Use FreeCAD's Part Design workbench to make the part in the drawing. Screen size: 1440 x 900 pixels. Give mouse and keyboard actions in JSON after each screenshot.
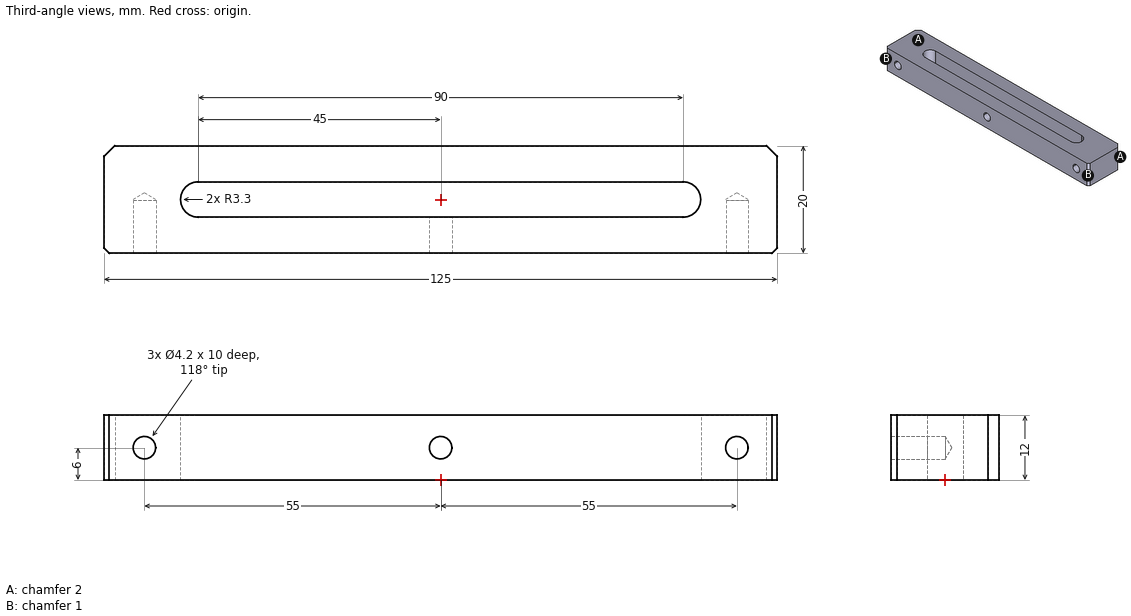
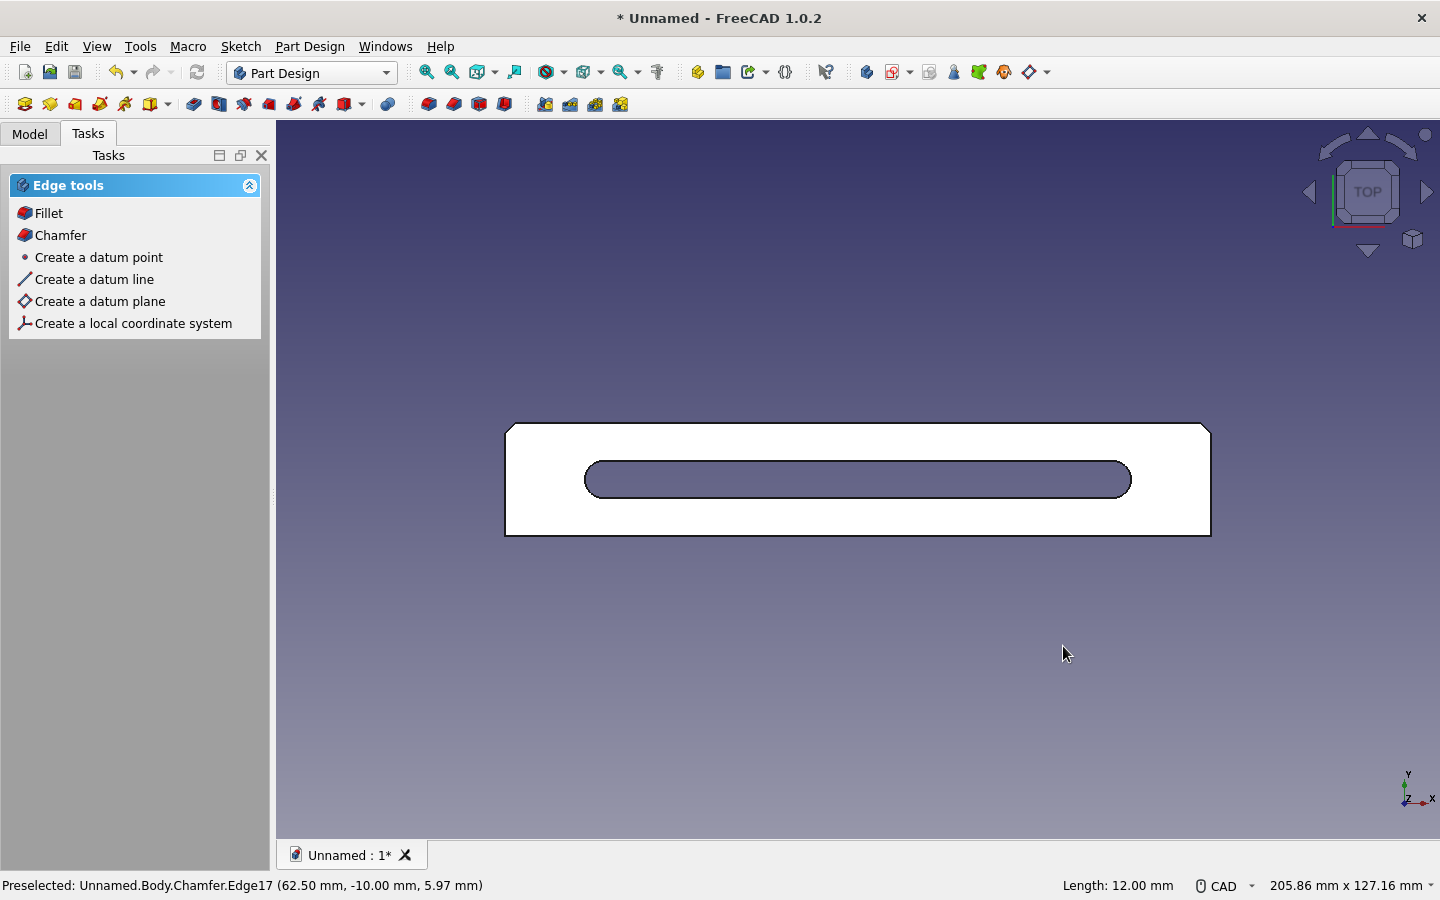
{"action": "key", "text": "1"}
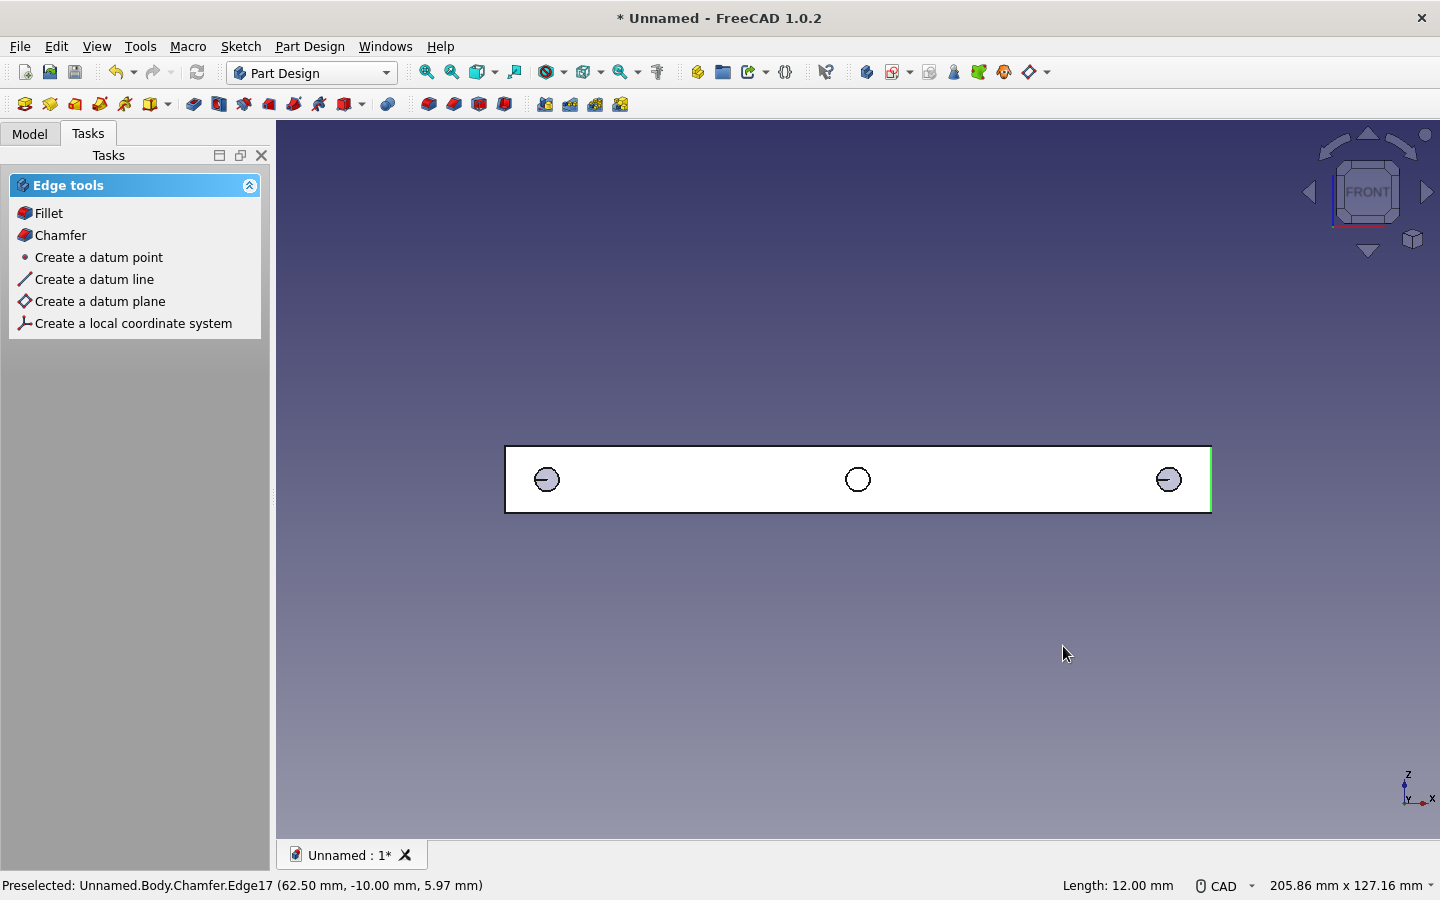
{"action": "left_click", "coordinate": [505, 479], "text": "ctrl"}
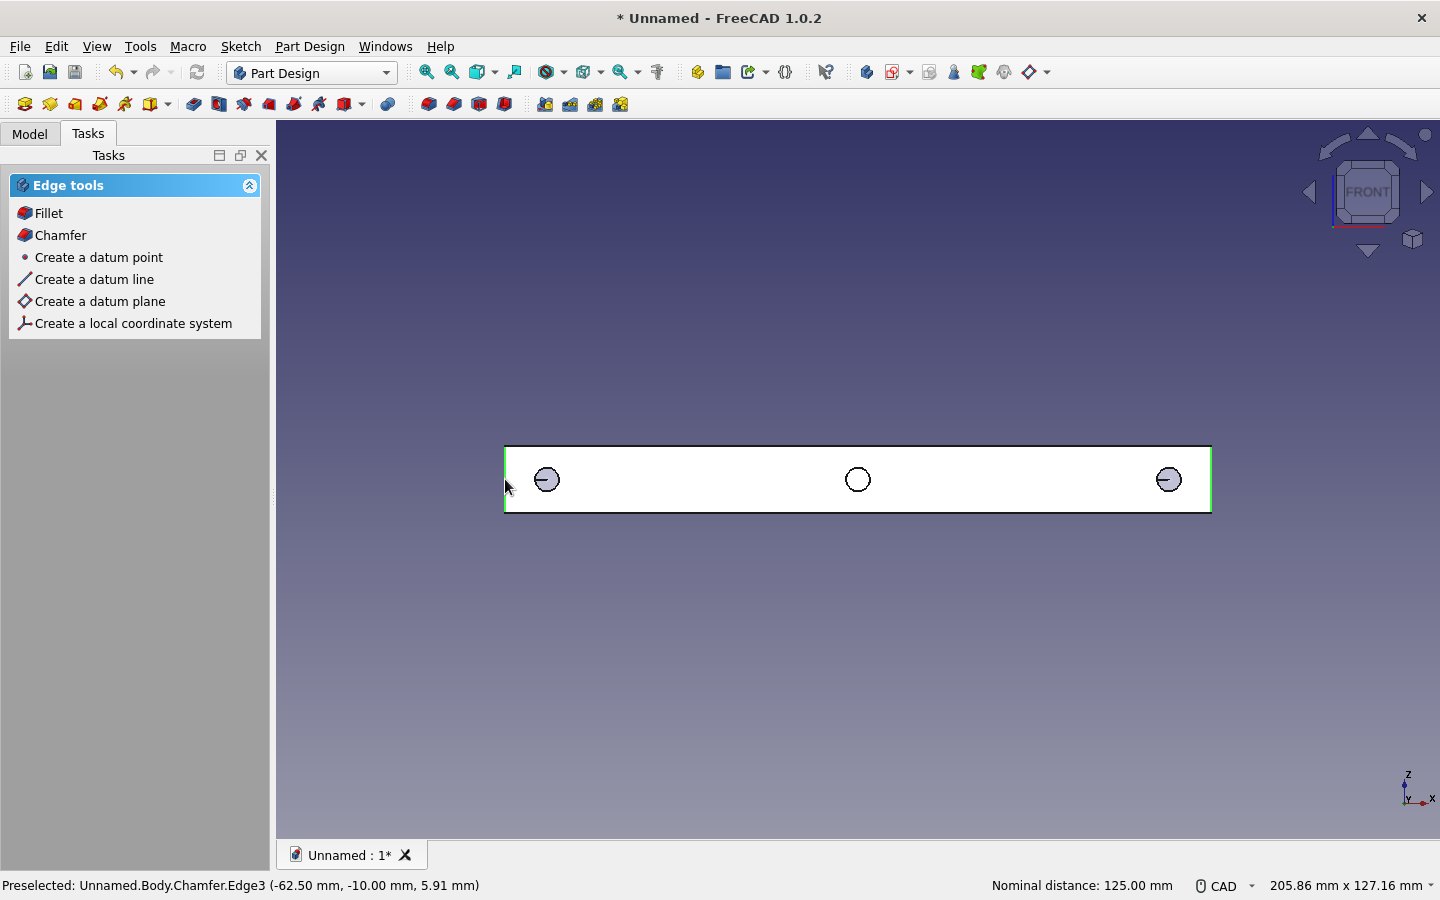
{"action": "left_click", "coordinate": [454, 104]}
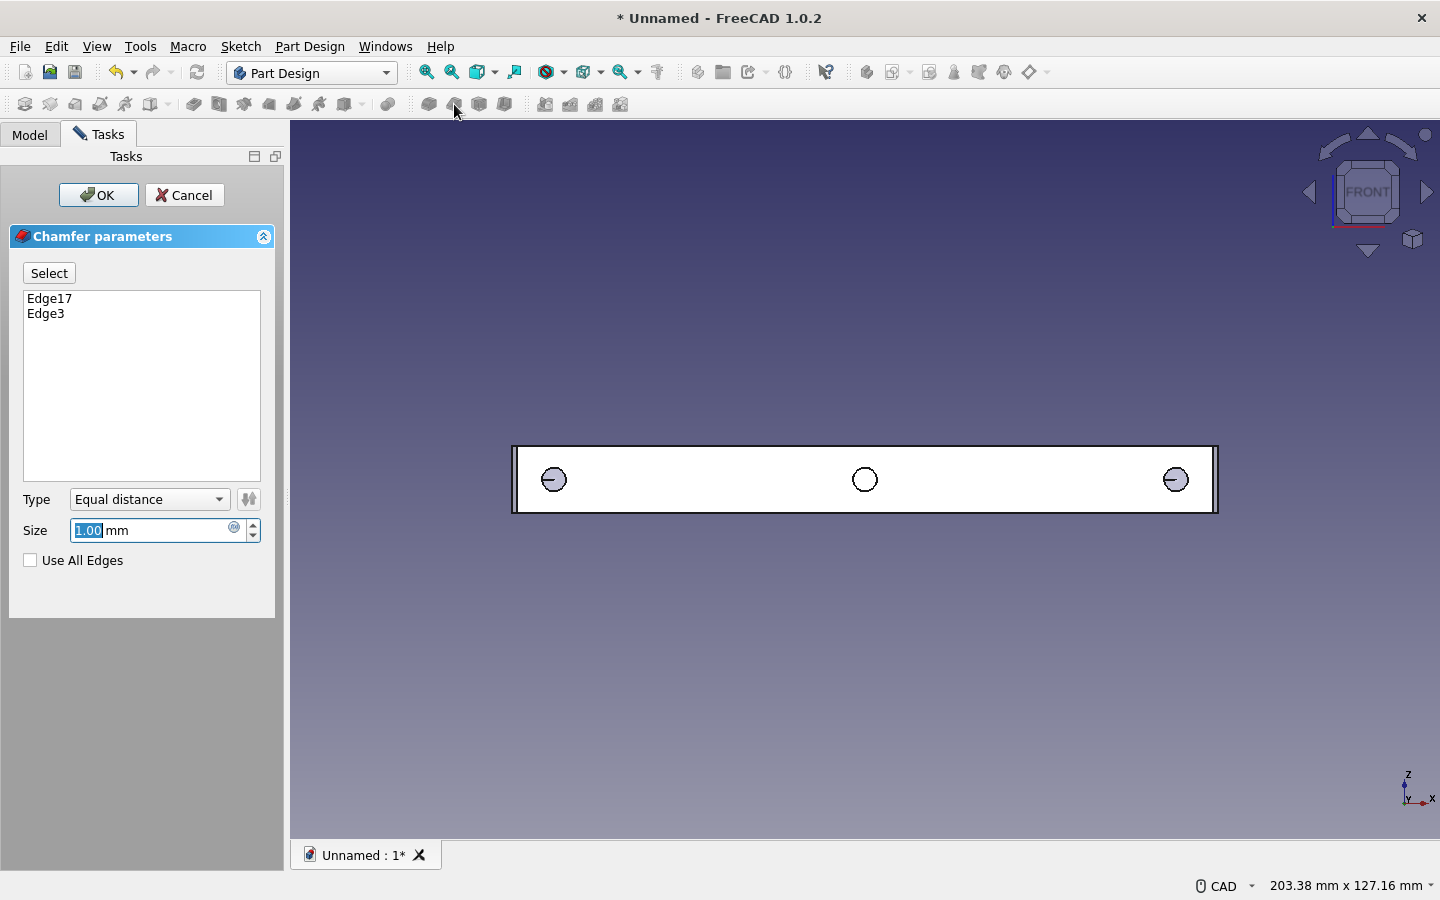
{"action": "type", "text": "1"}
{"action": "key", "text": "Tab"}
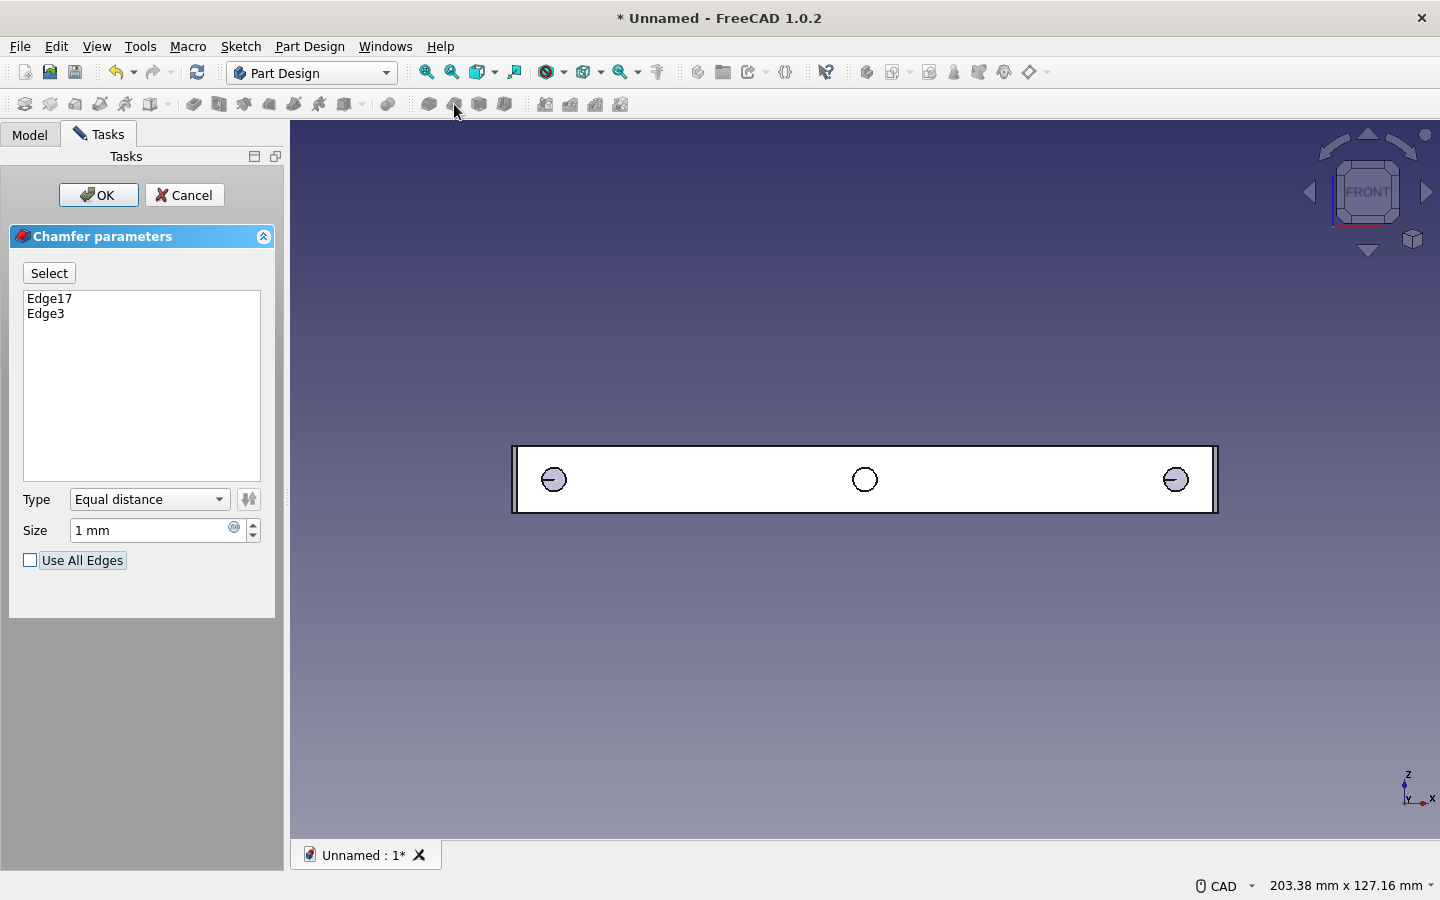
{"action": "left_click", "coordinate": [99, 195]}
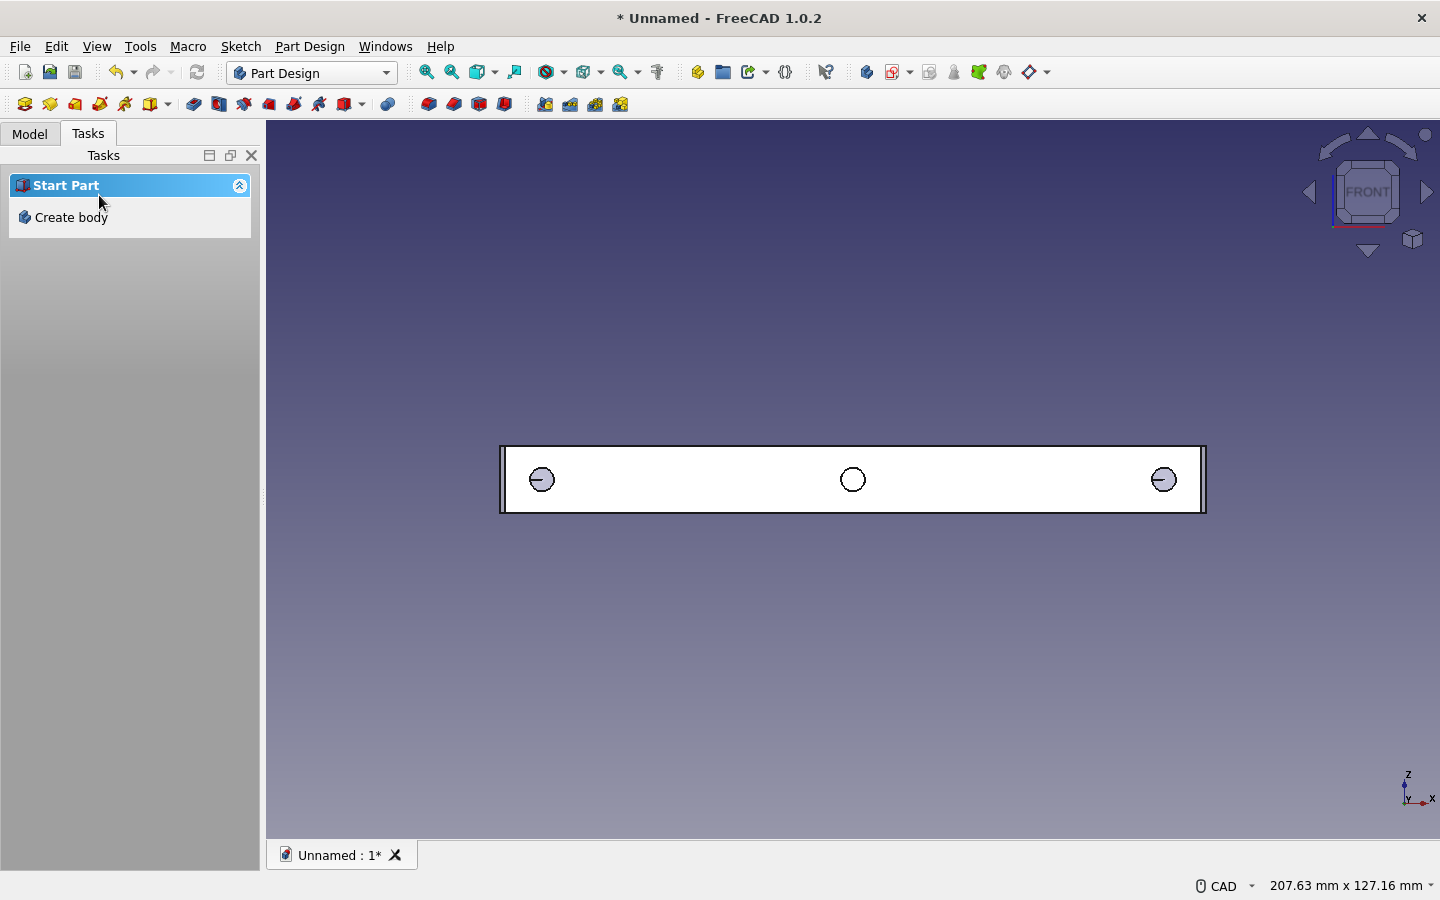
{"action": "key", "text": "0"}